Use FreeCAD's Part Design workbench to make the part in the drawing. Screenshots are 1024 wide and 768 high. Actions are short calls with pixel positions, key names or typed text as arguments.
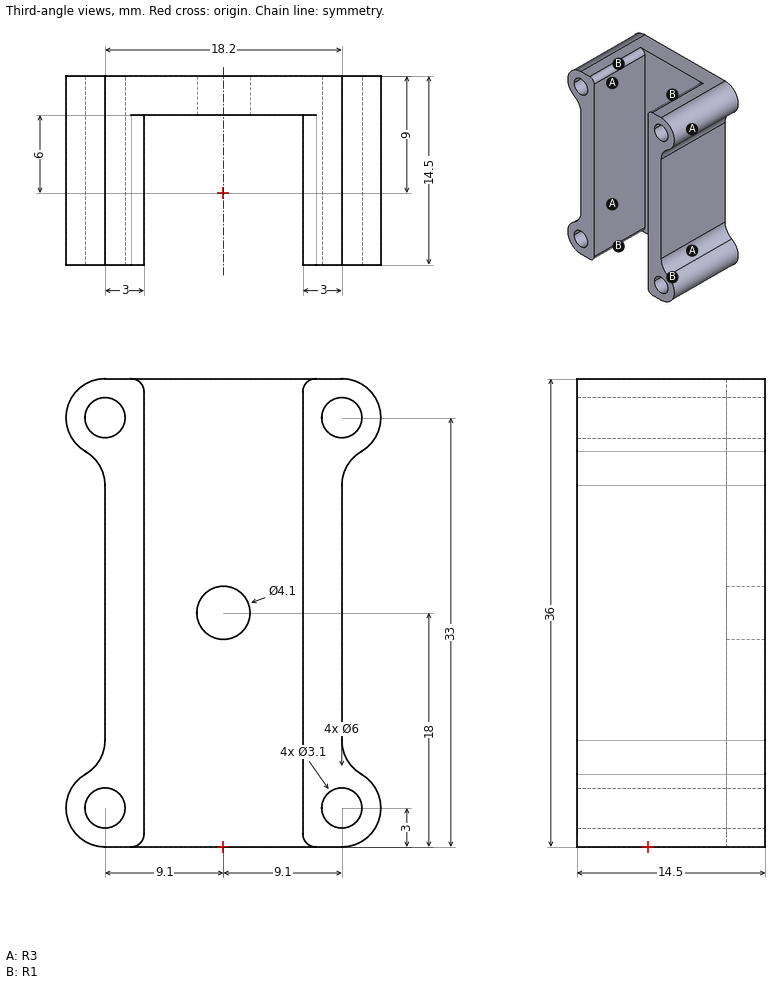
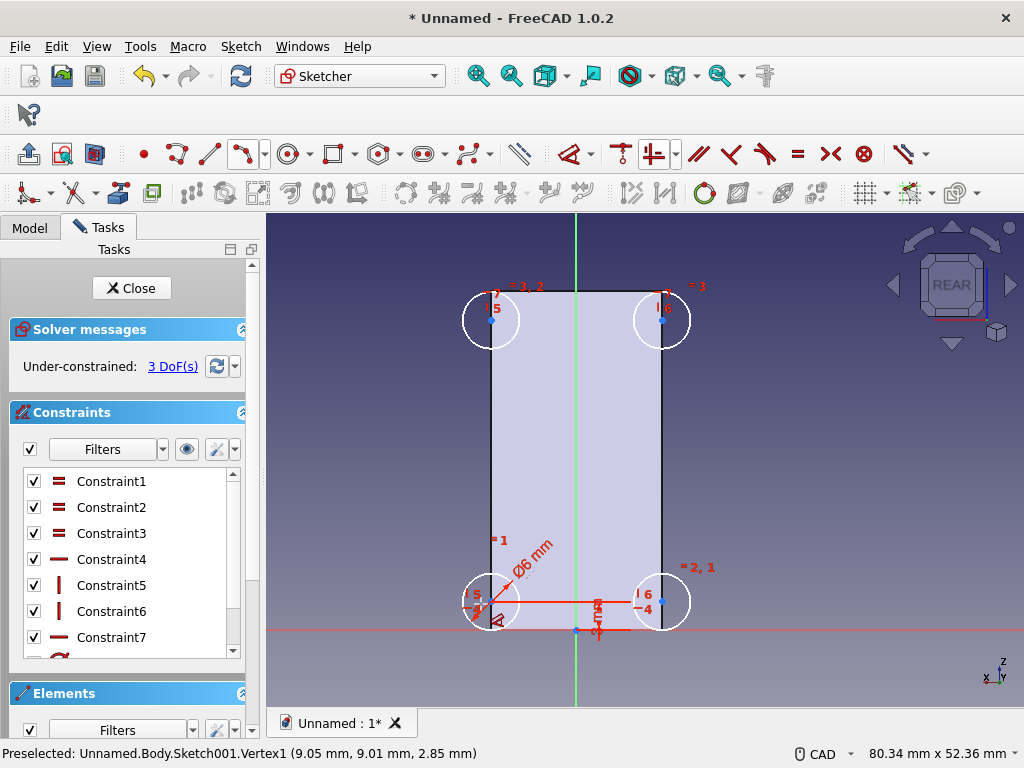
click(491, 320)
click(457, 475)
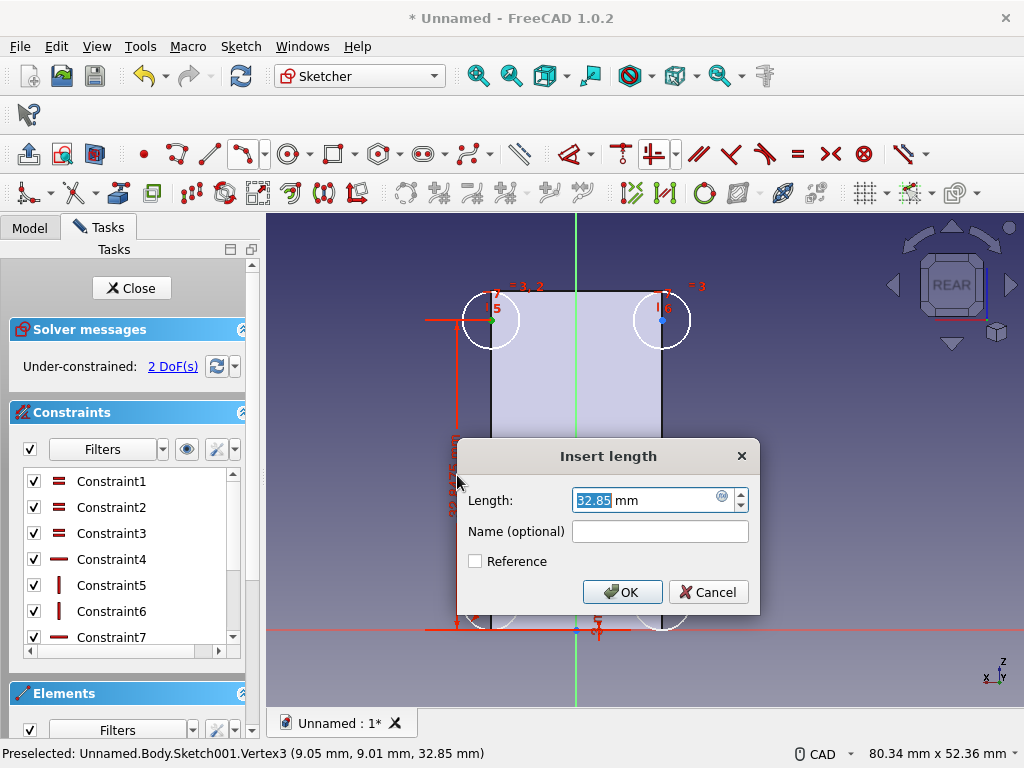
text(33)
key(Return)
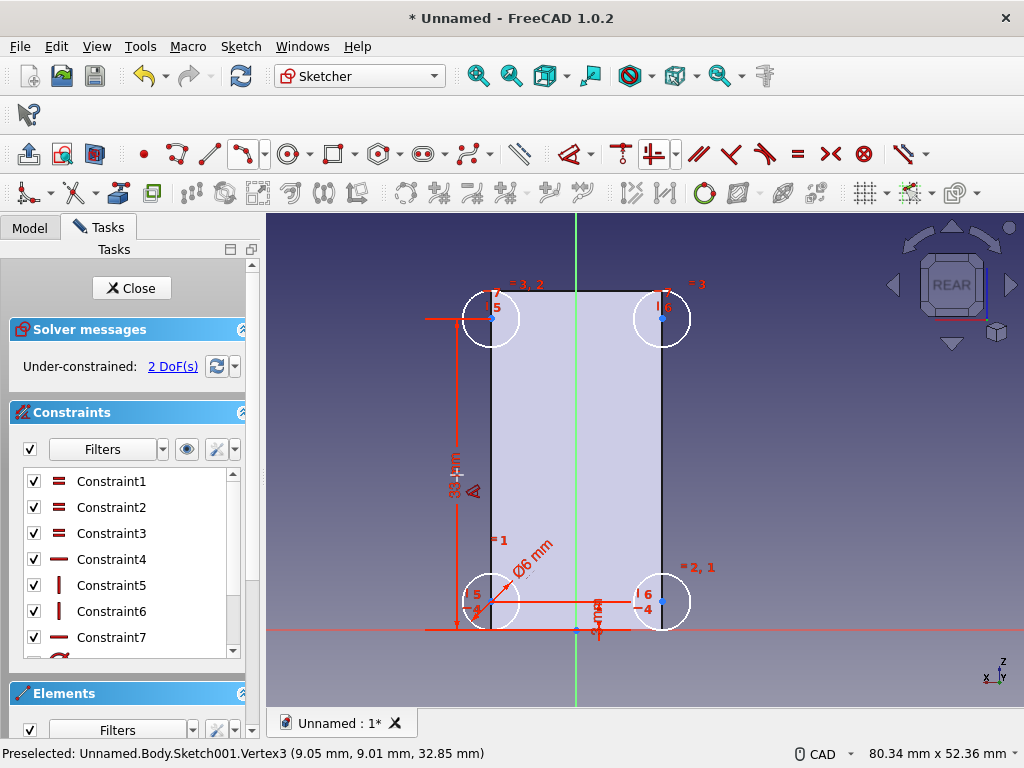
click(491, 602)
click(534, 664)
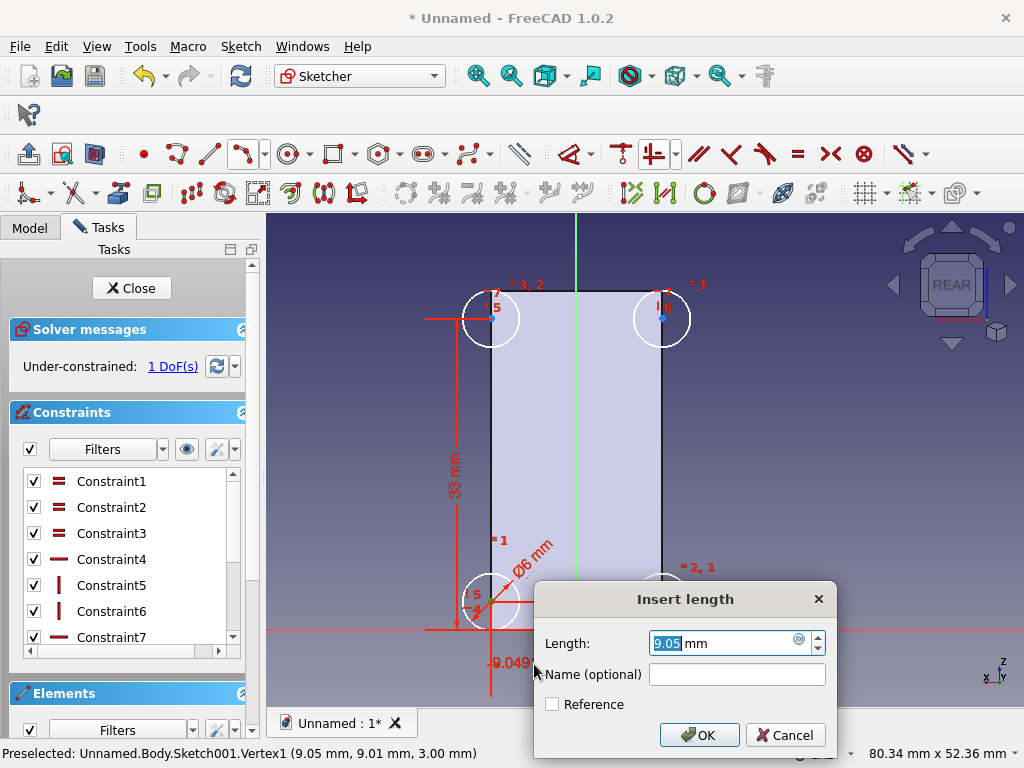
text(9.1)
key(Return)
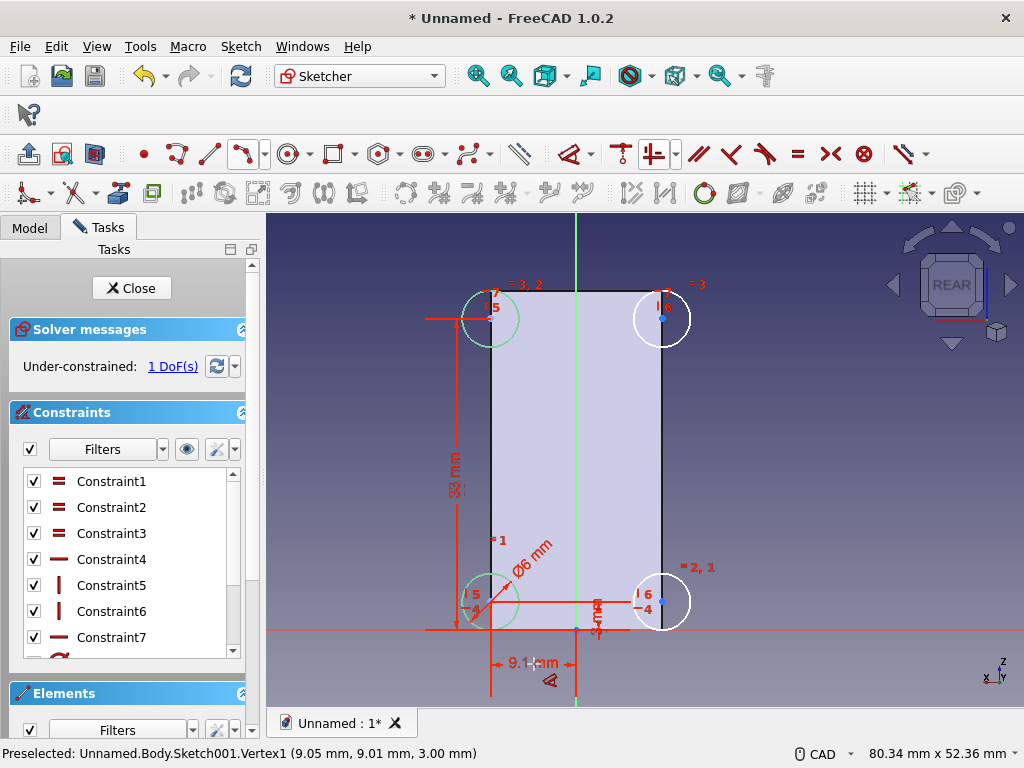
click(662, 602)
click(619, 664)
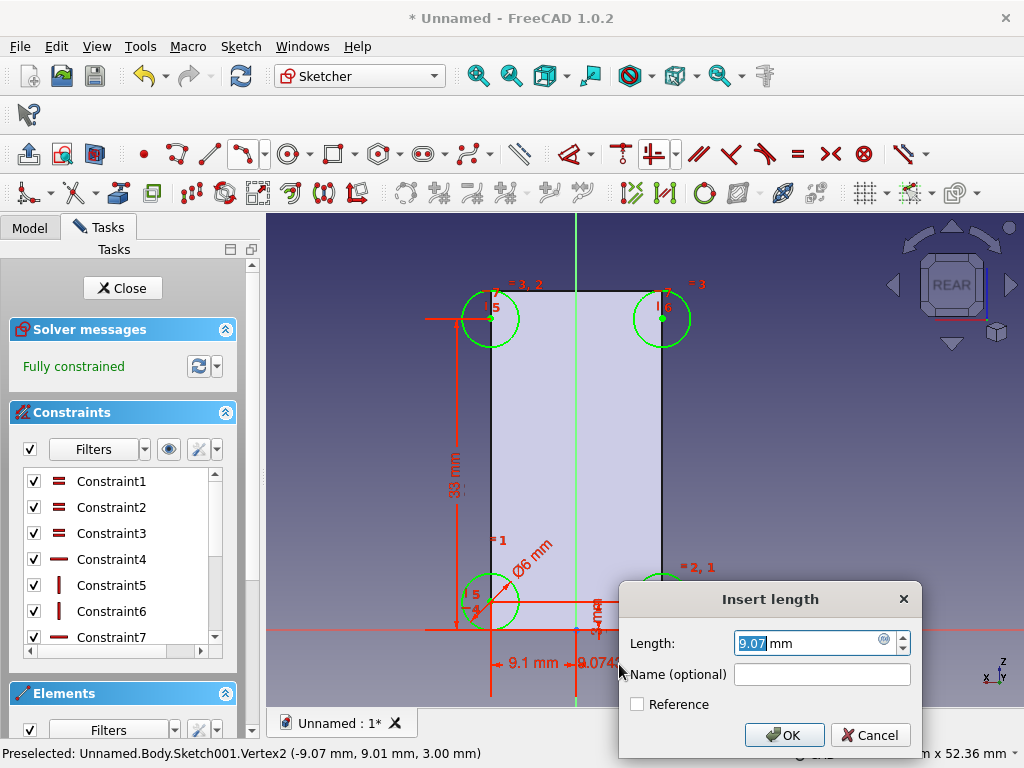
text(9.1)
key(Return)
key(Escape)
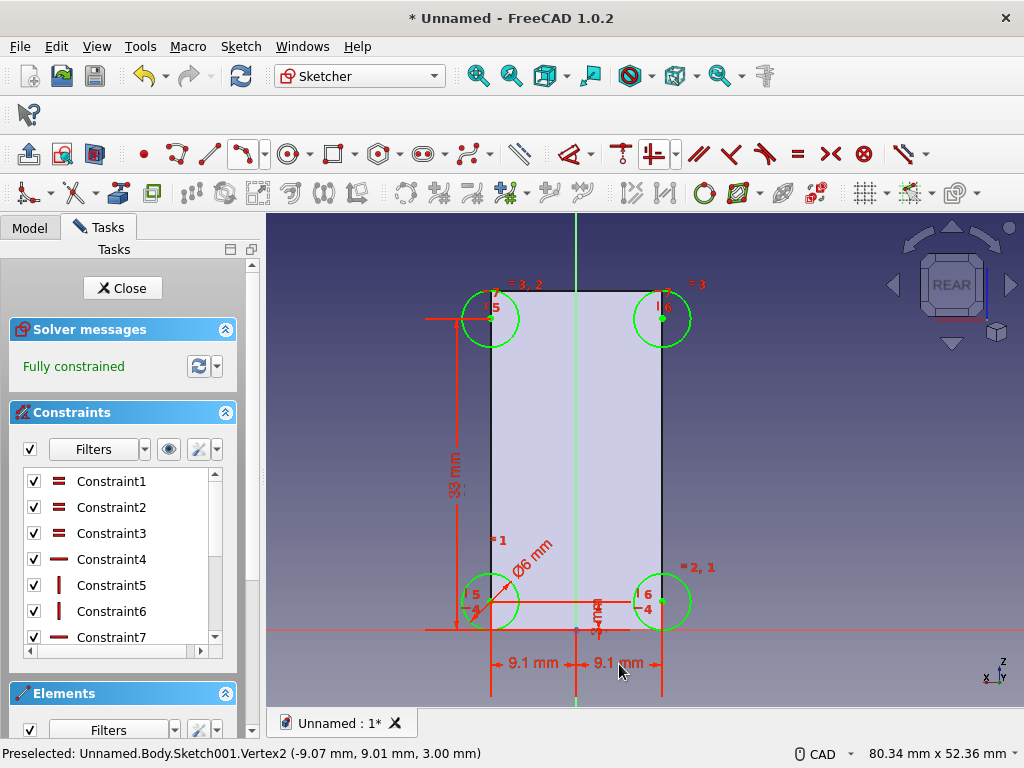
click(123, 288)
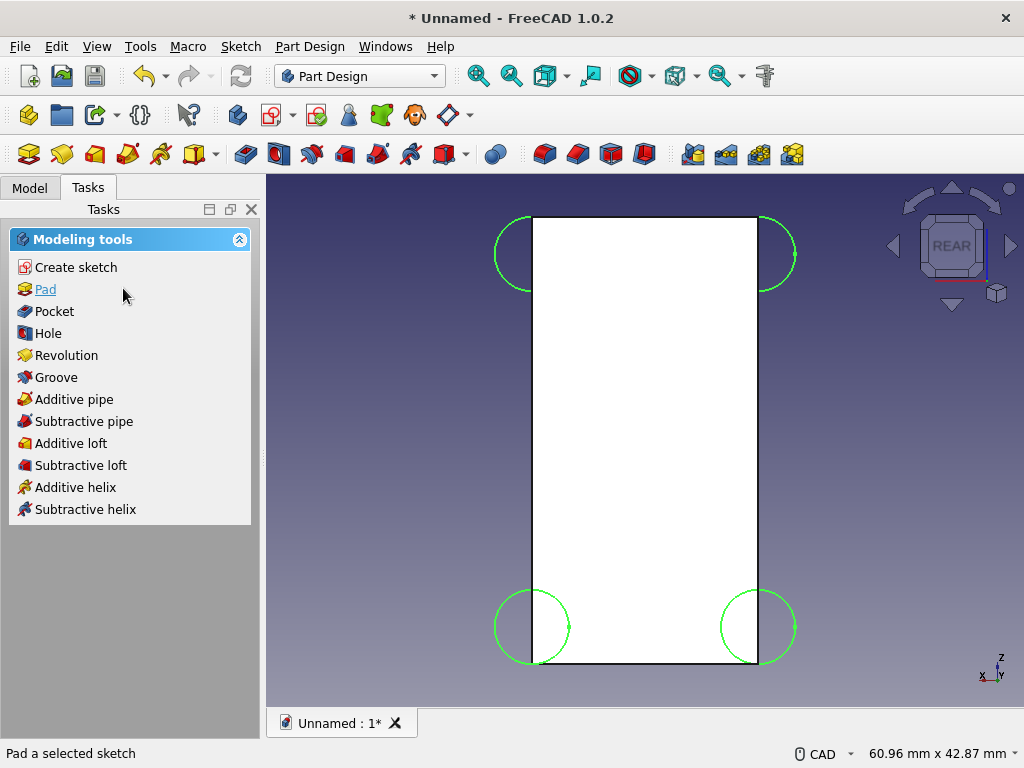
click(29, 154)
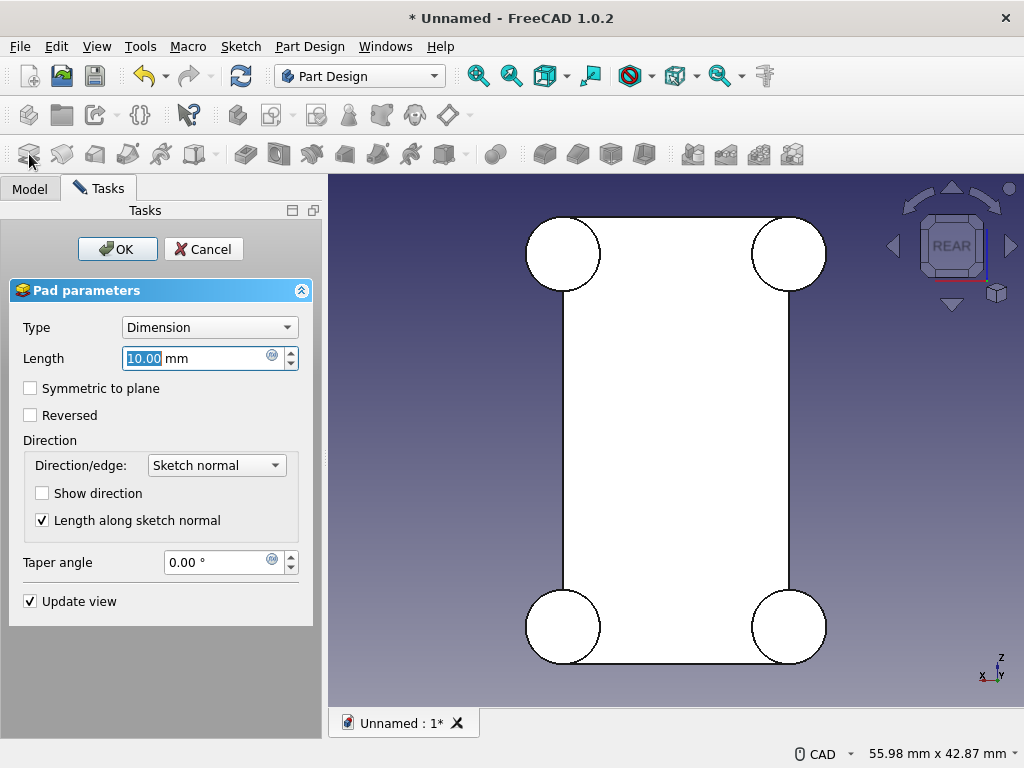
text(14.5)
key(Tab)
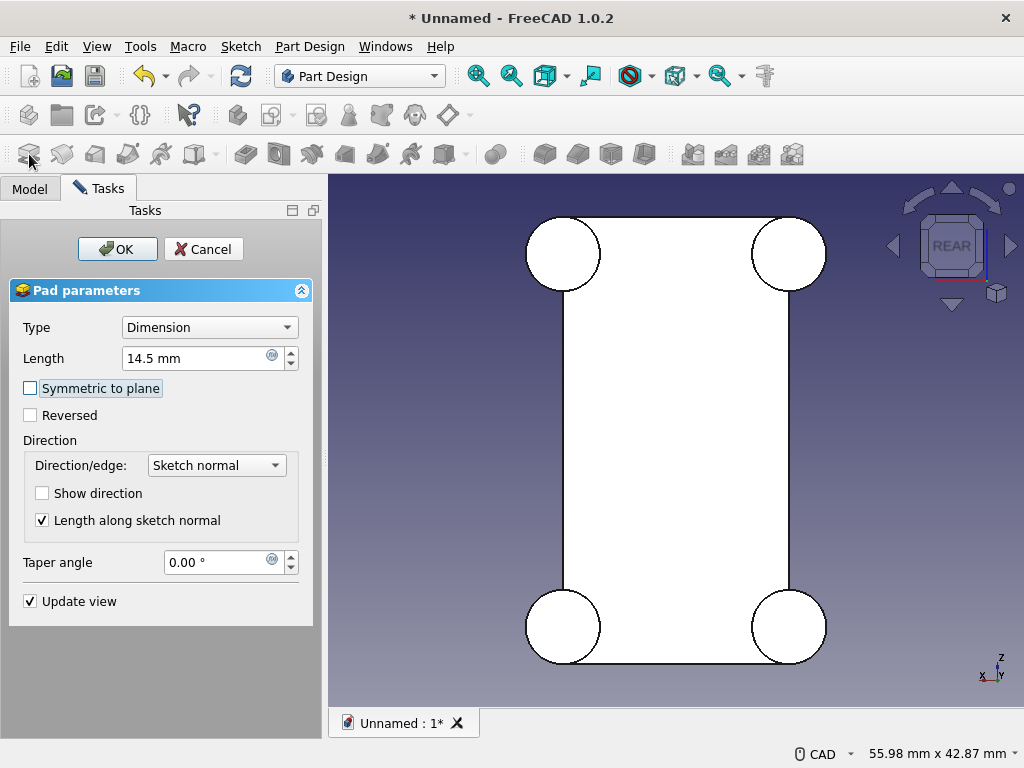
click(31, 415)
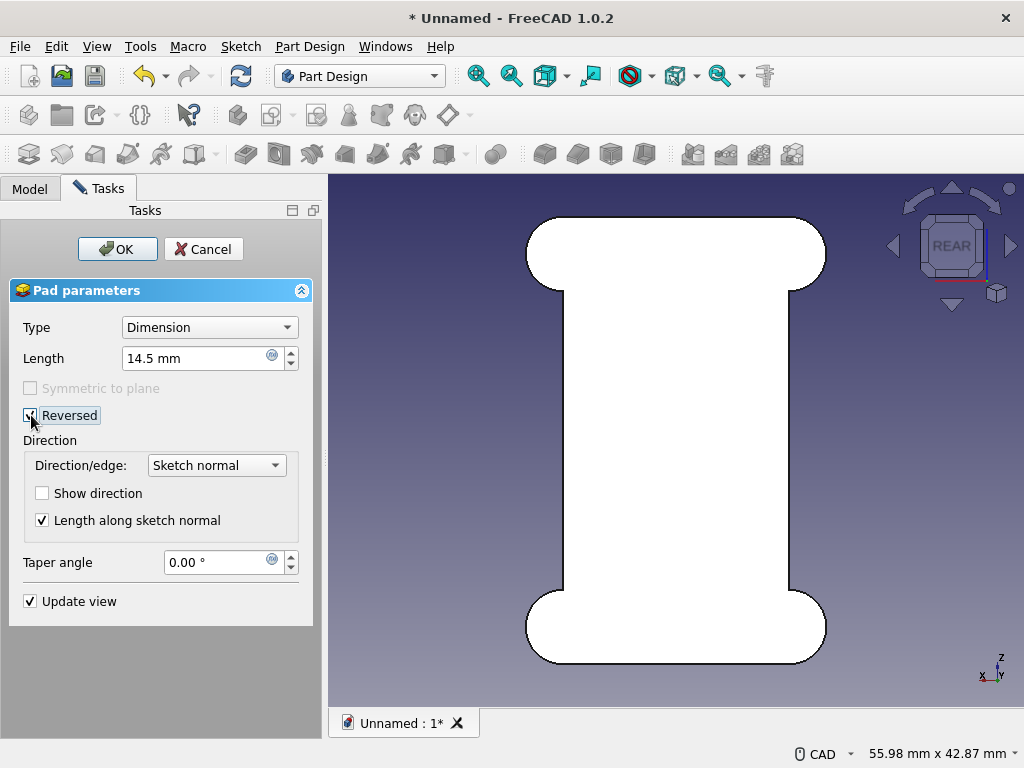
click(118, 249)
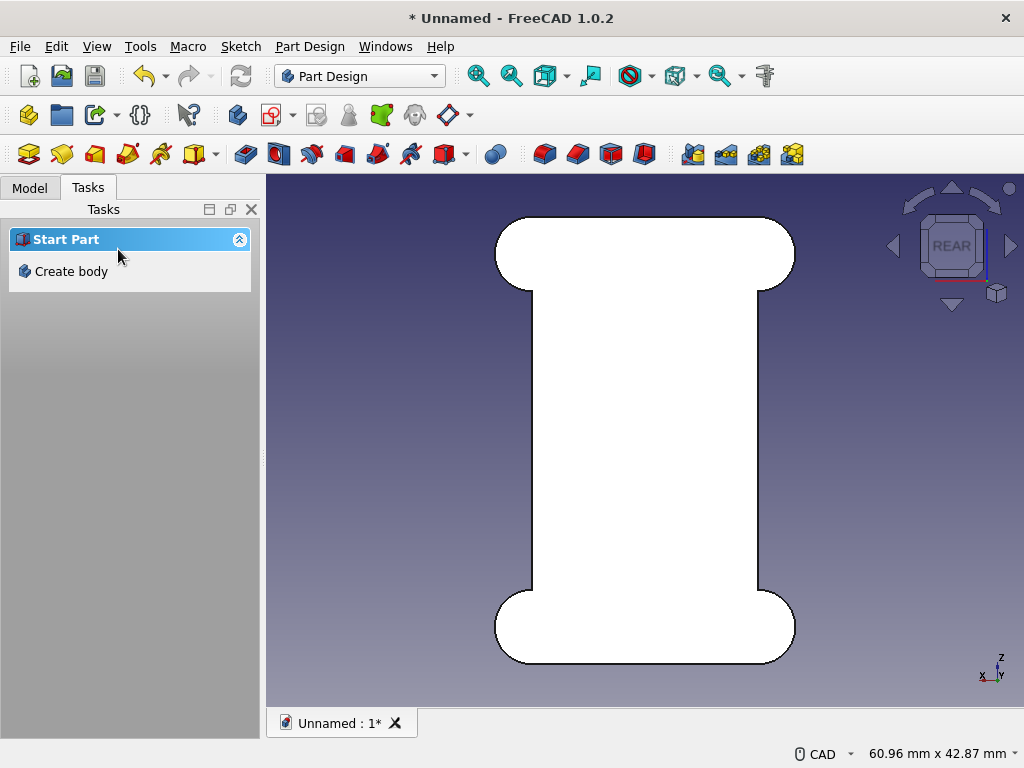
click(645, 376)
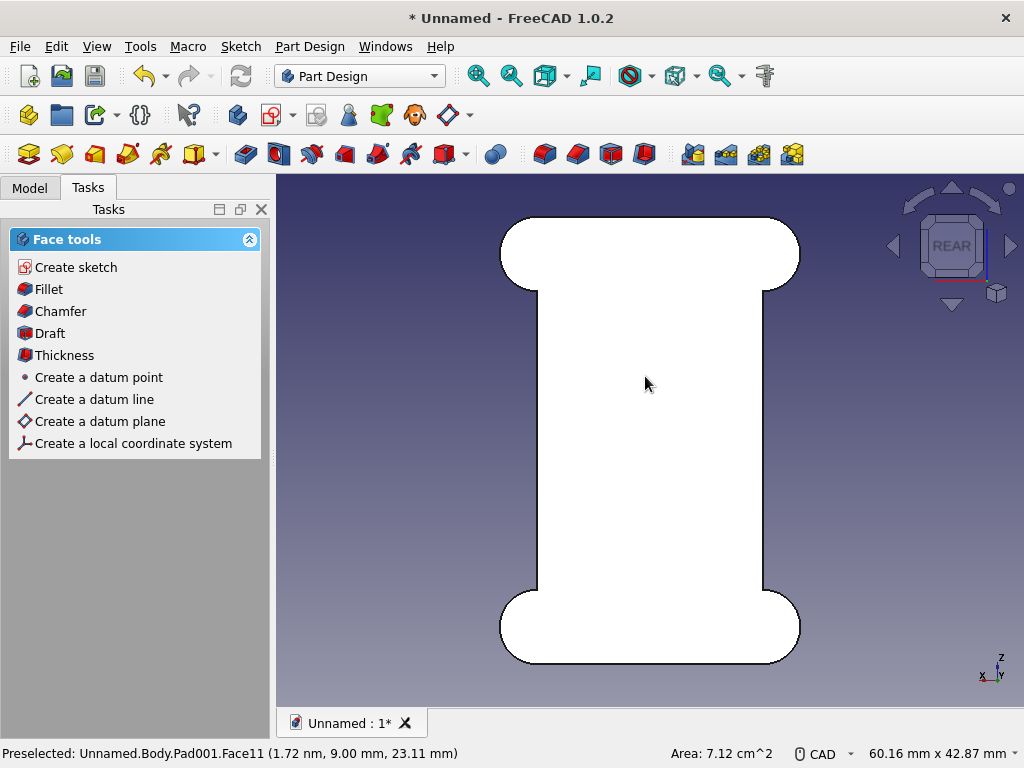
click(270, 116)